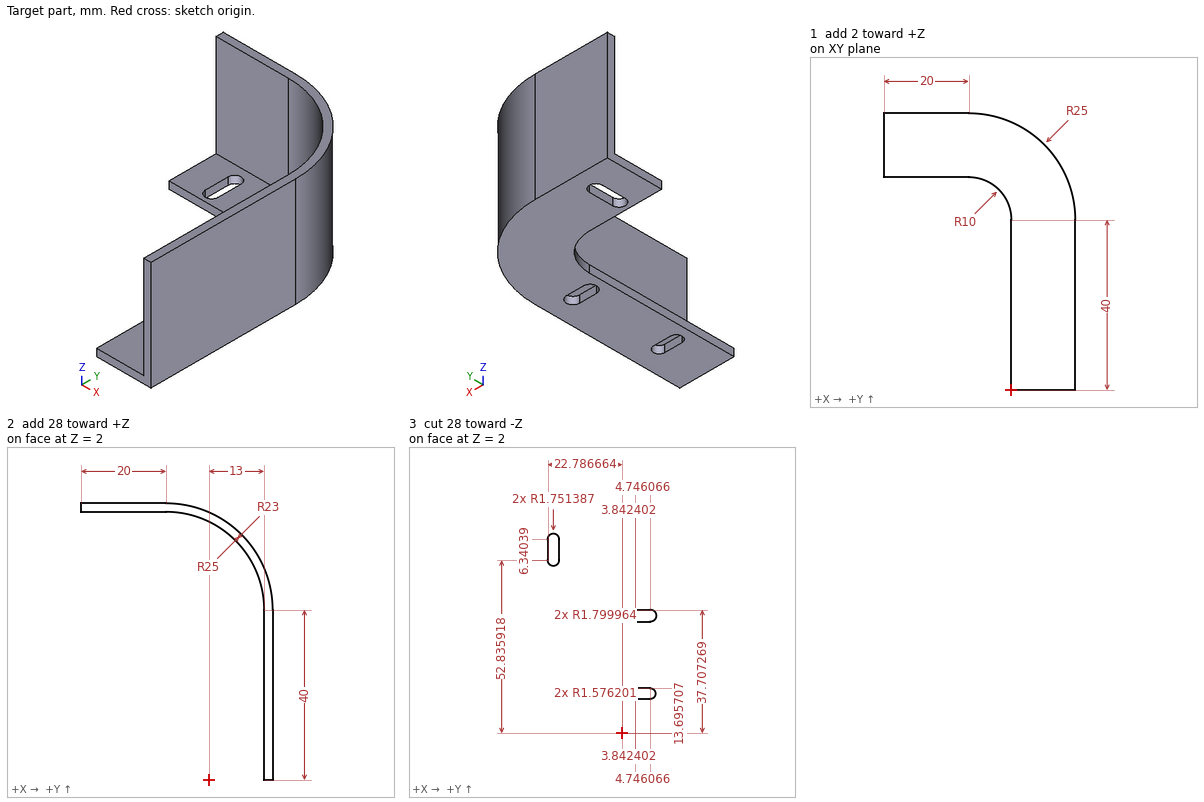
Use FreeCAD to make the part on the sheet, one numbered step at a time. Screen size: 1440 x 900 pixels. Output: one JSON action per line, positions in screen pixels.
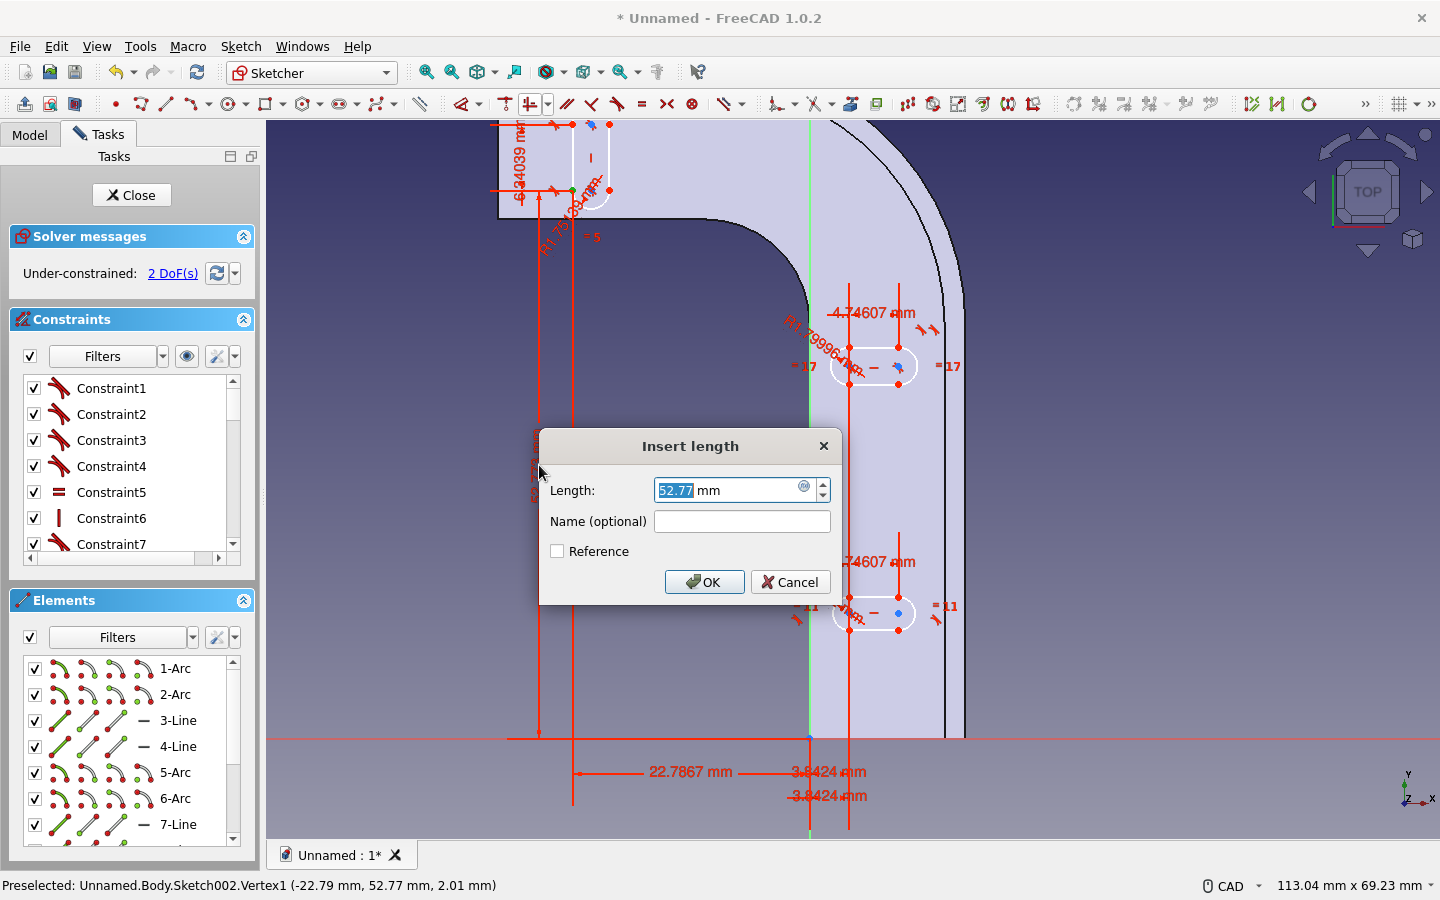
{"action": "type", "text": "52.835918"}
{"action": "key", "text": "Return"}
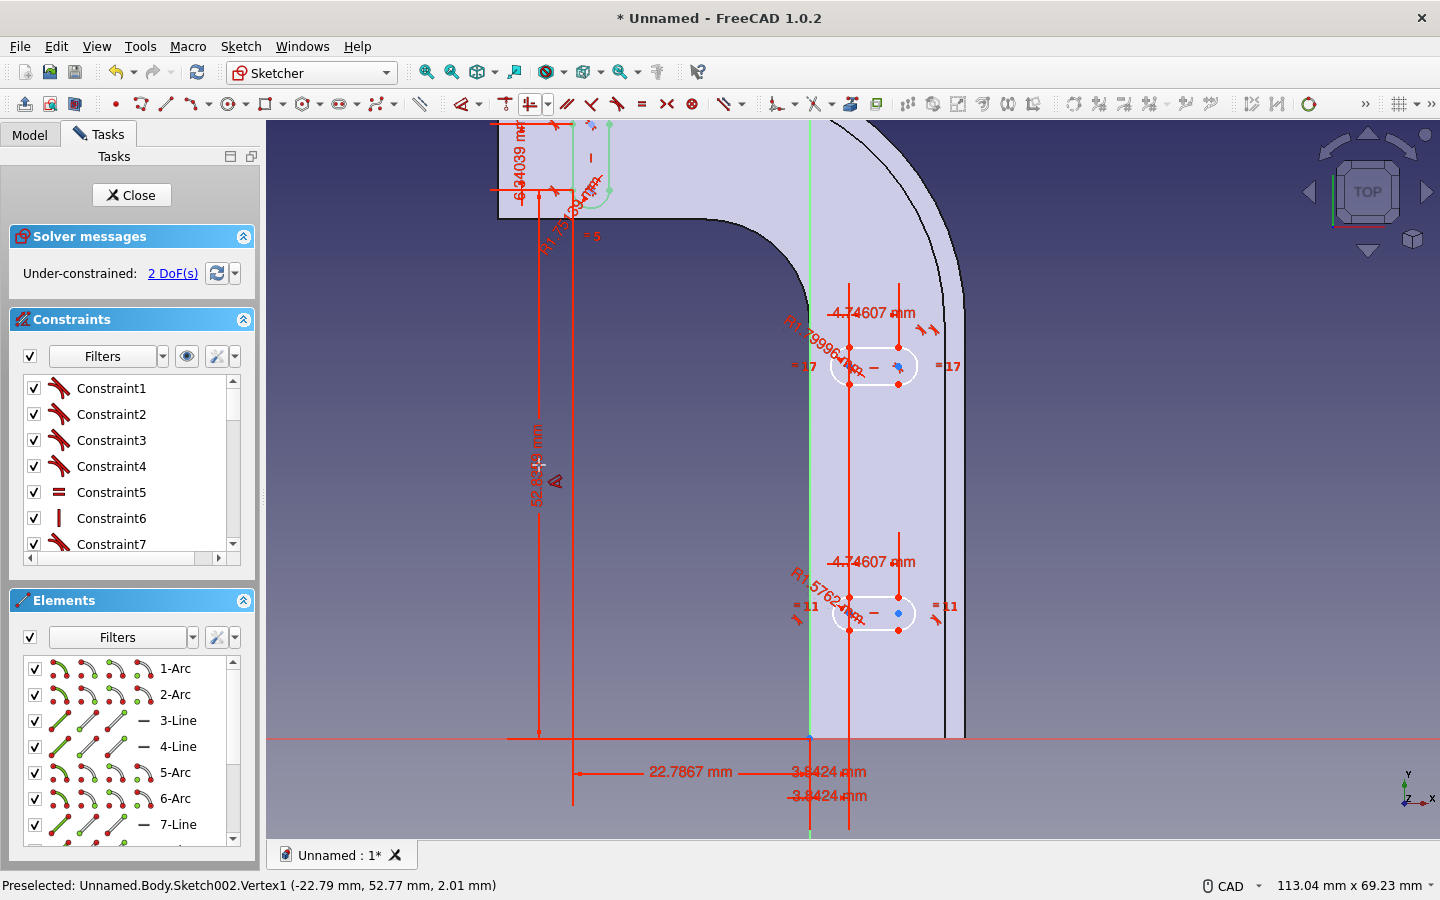
{"action": "left_click", "coordinate": [849, 597]}
{"action": "left_click", "coordinate": [883, 668]}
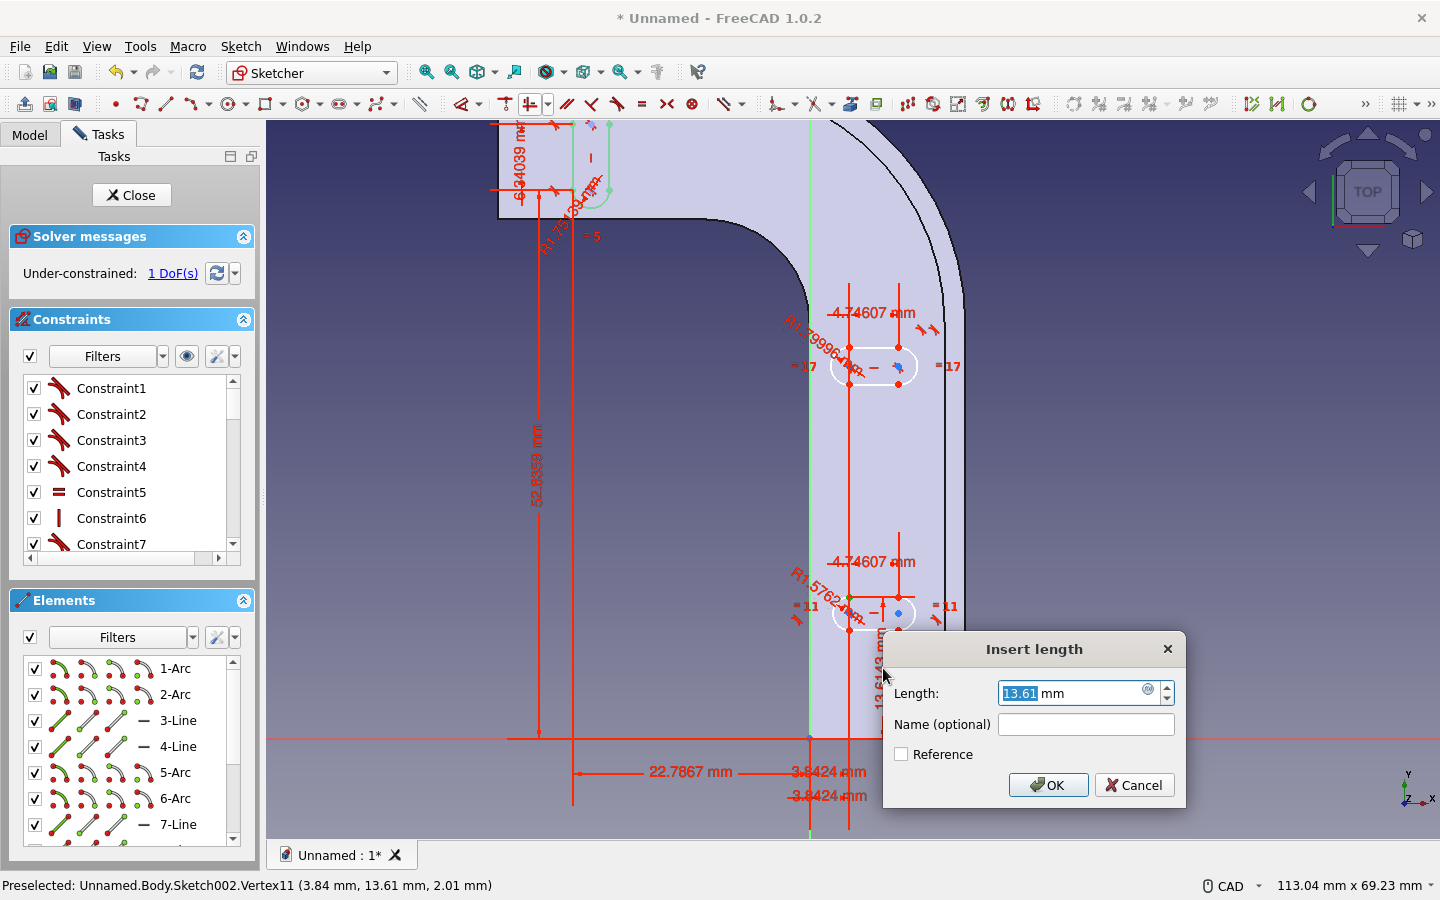
{"action": "type", "text": "13.695707"}
{"action": "key", "text": "Return"}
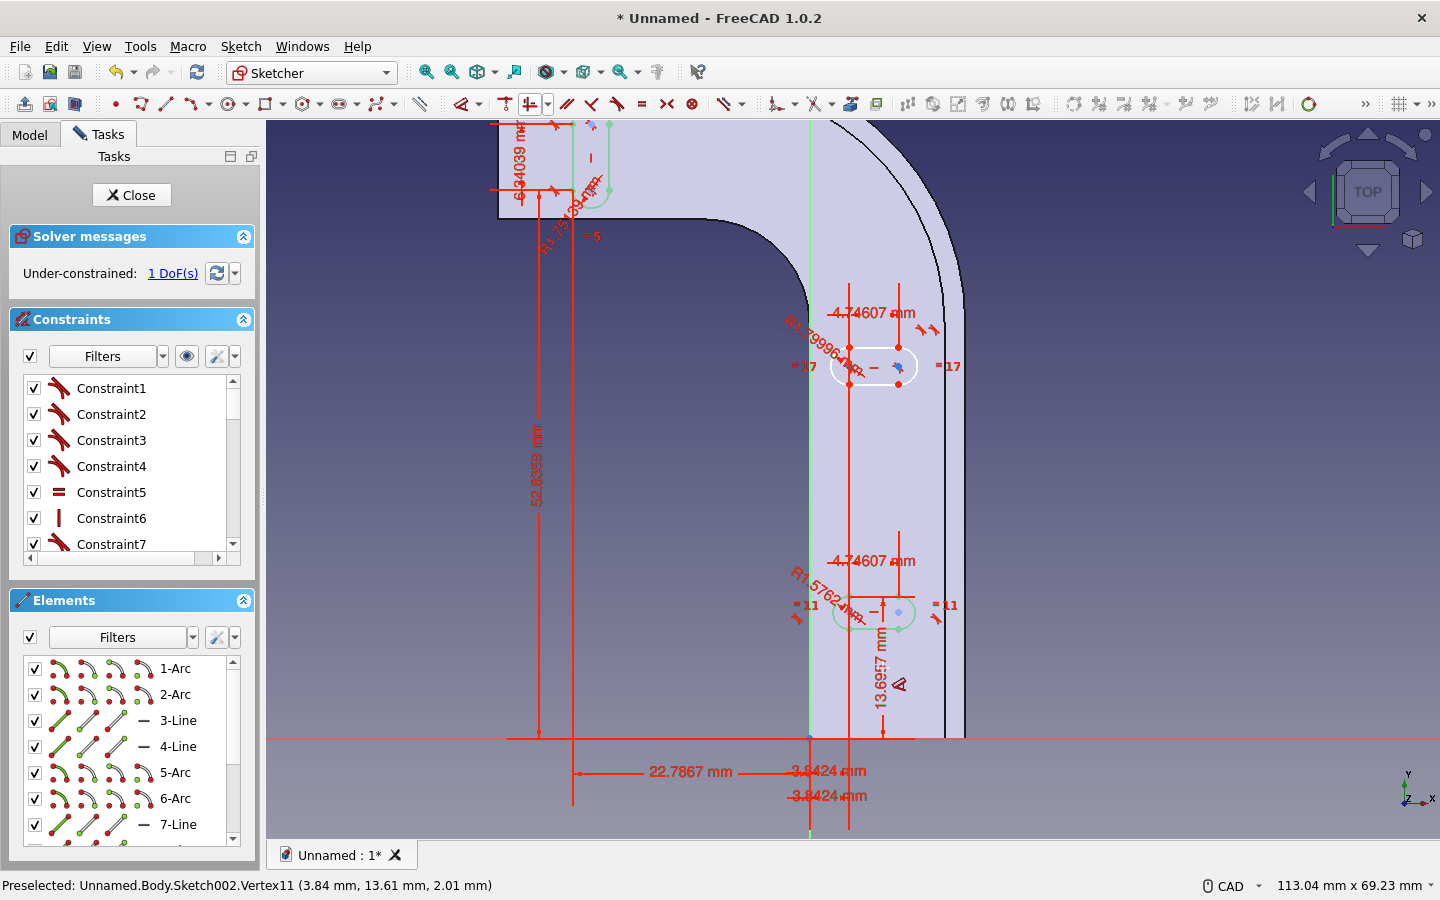
{"action": "left_click", "coordinate": [849, 348]}
{"action": "left_click", "coordinate": [883, 543]}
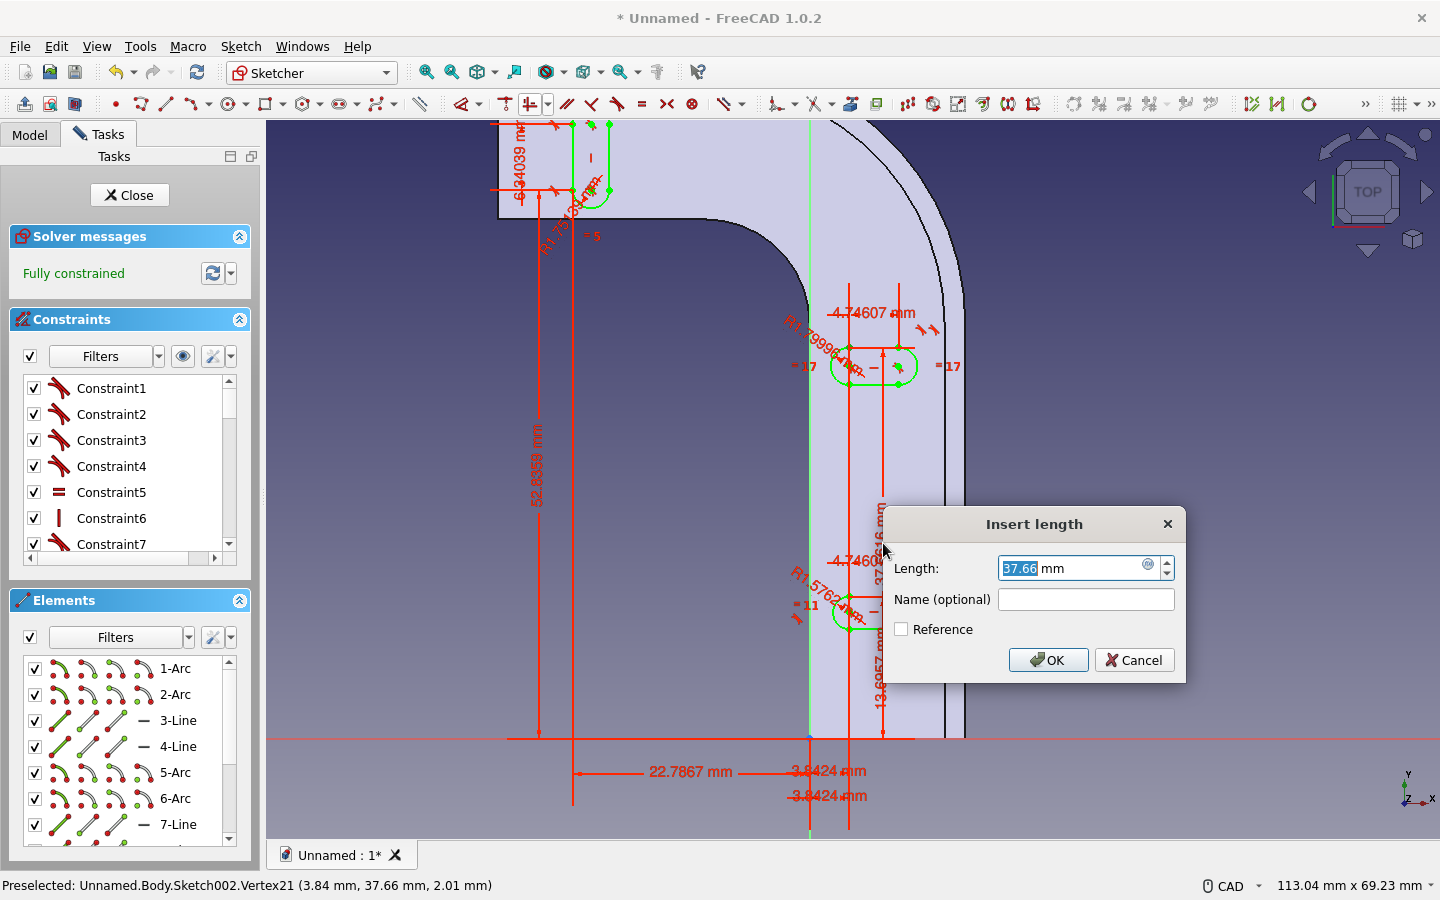
{"action": "type", "text": "37.707269"}
{"action": "key", "text": "Return"}
{"action": "key", "text": "Escape"}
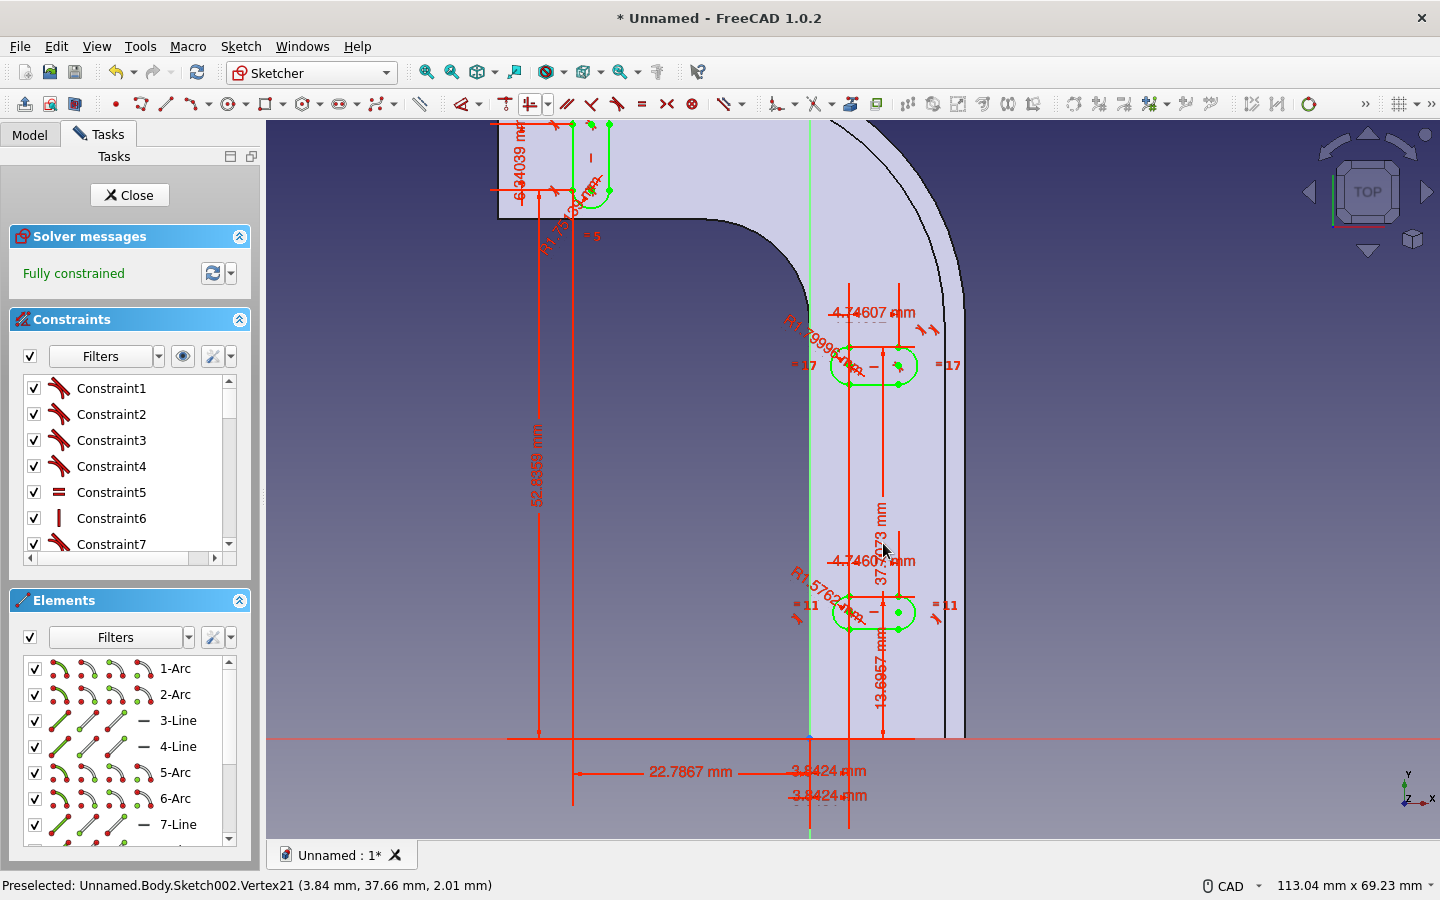
{"action": "left_click", "coordinate": [130, 195]}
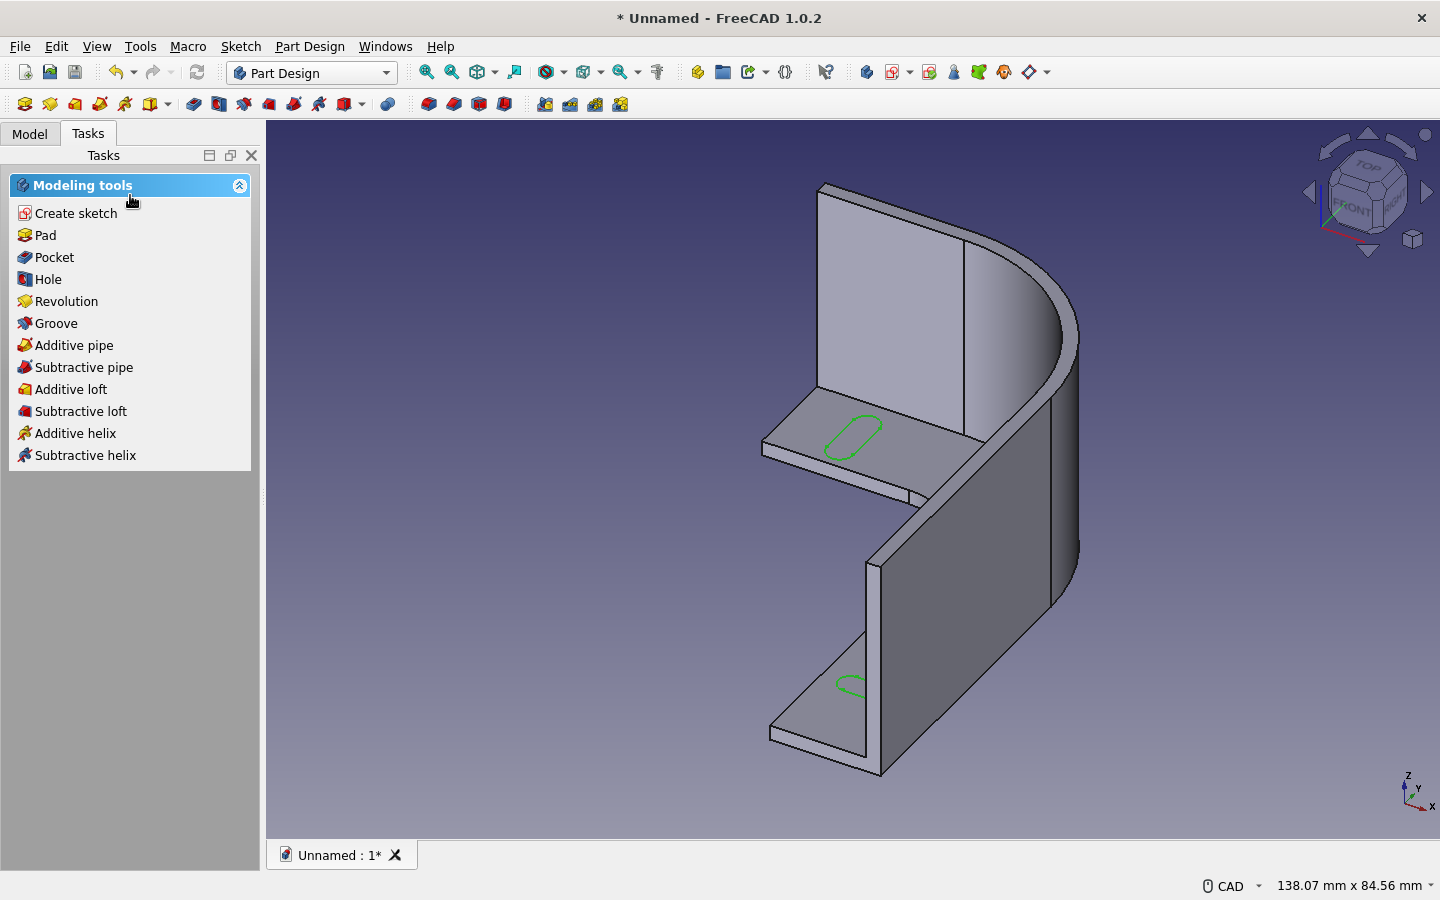
{"action": "left_click", "coordinate": [194, 104]}